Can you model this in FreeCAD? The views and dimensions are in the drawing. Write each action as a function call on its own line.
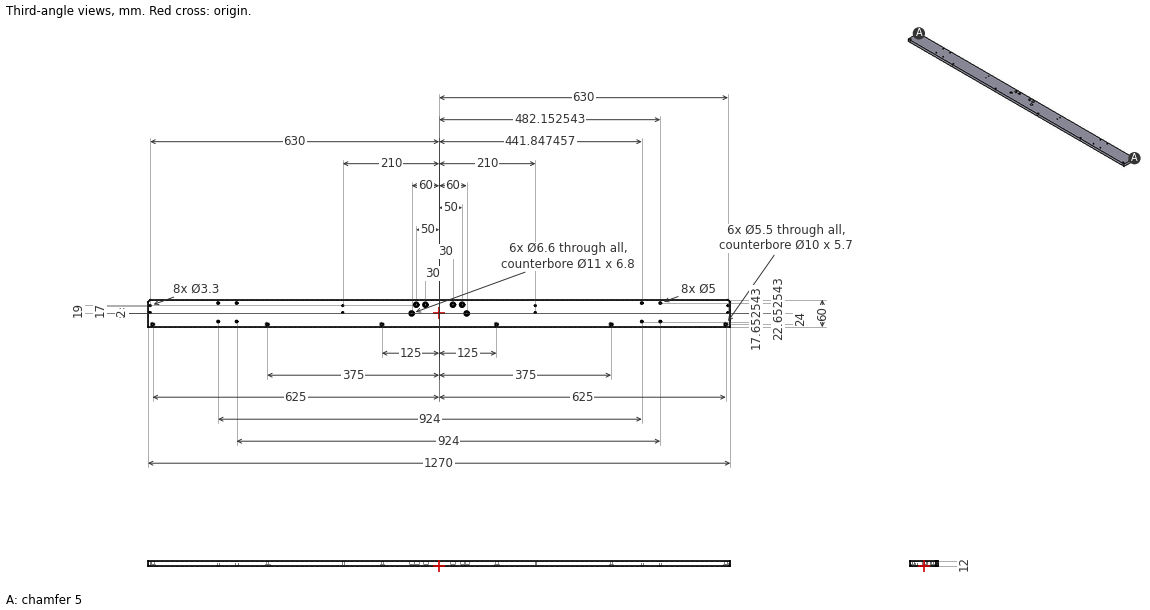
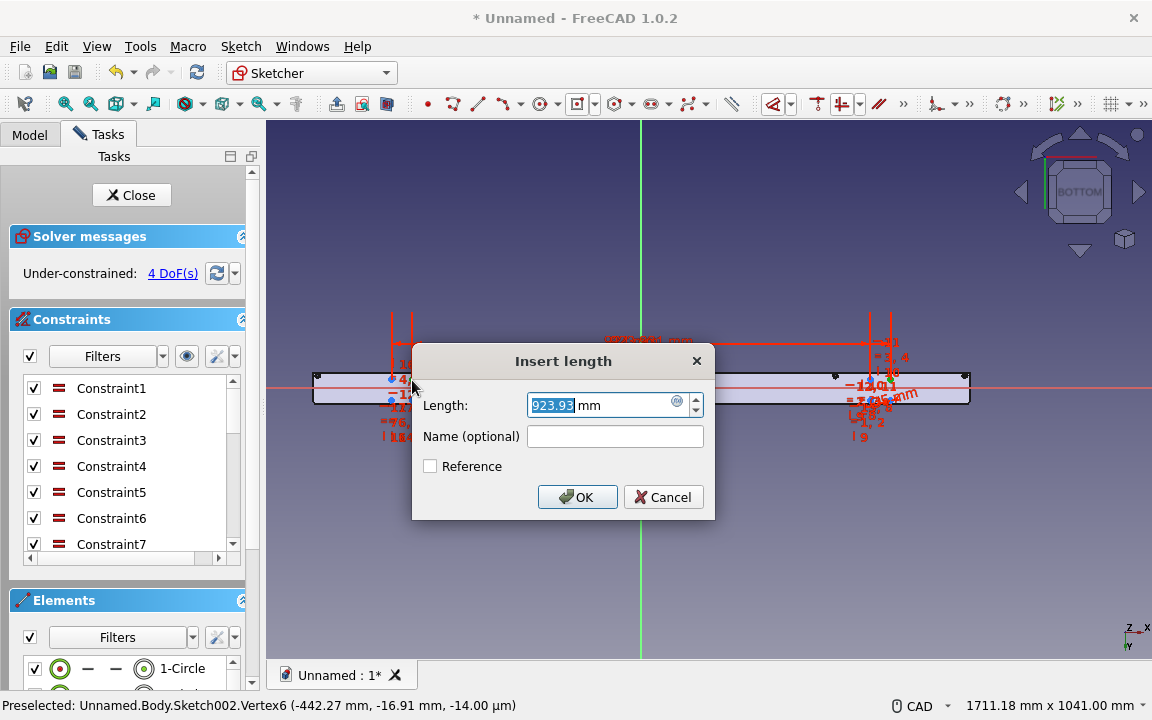
text(924)
key(Return)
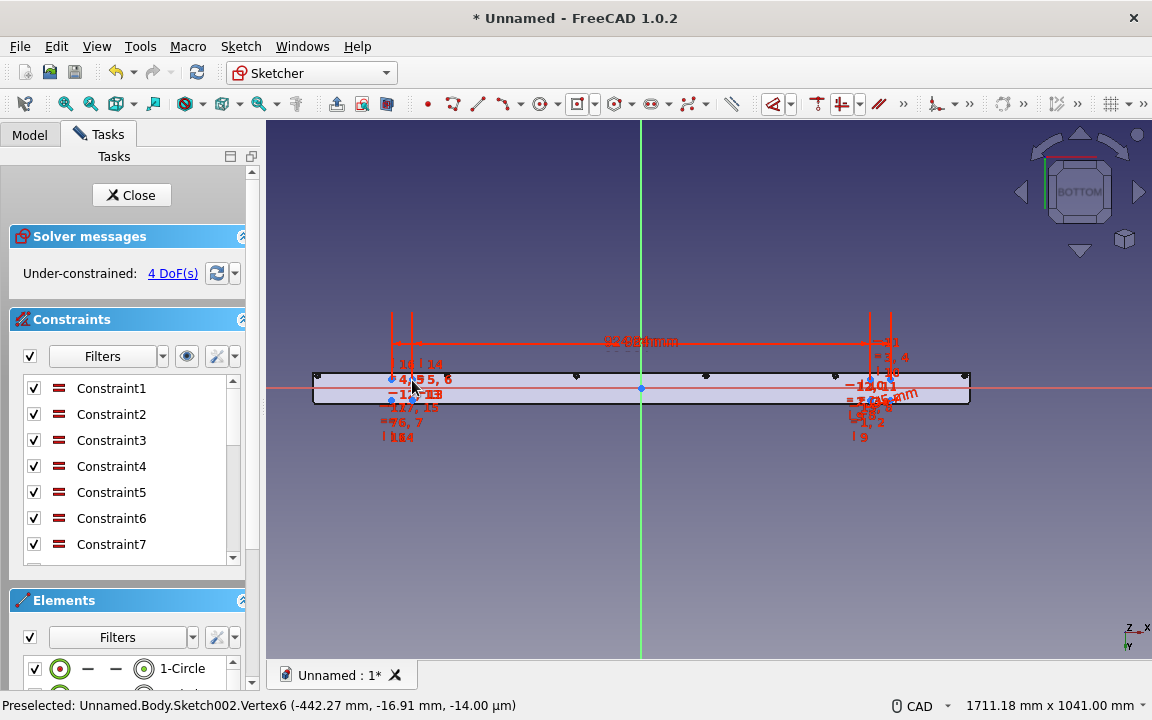
scroll(891, 401, up, 7)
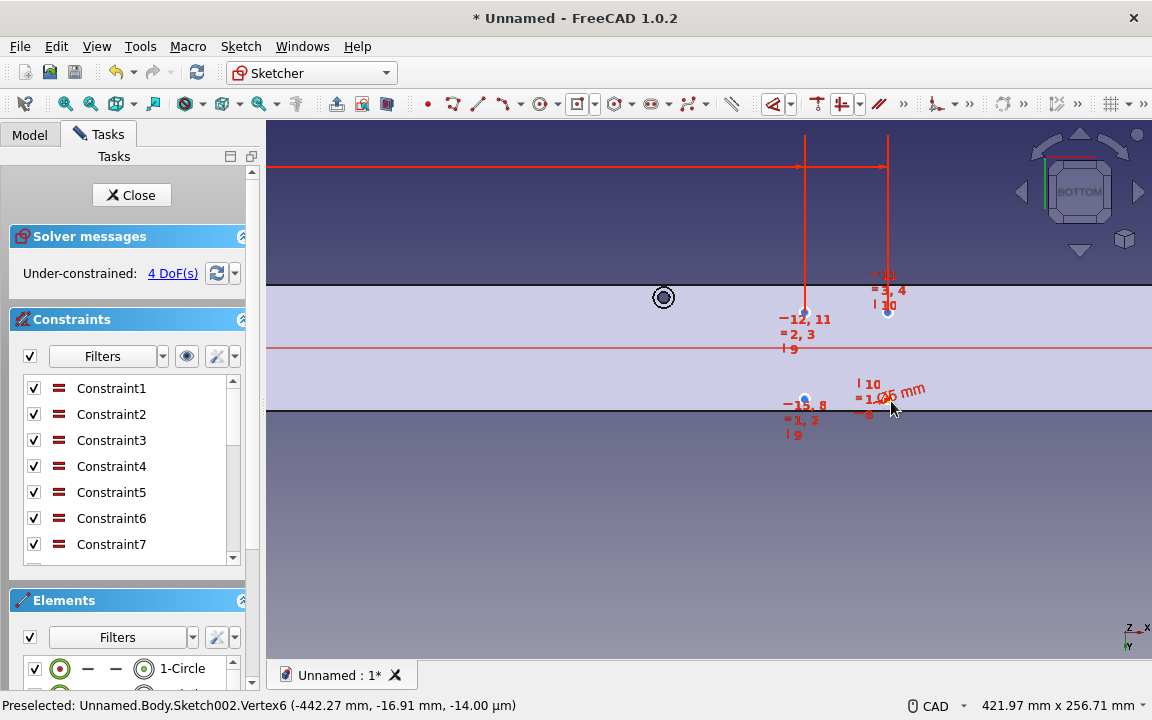
click(888, 399)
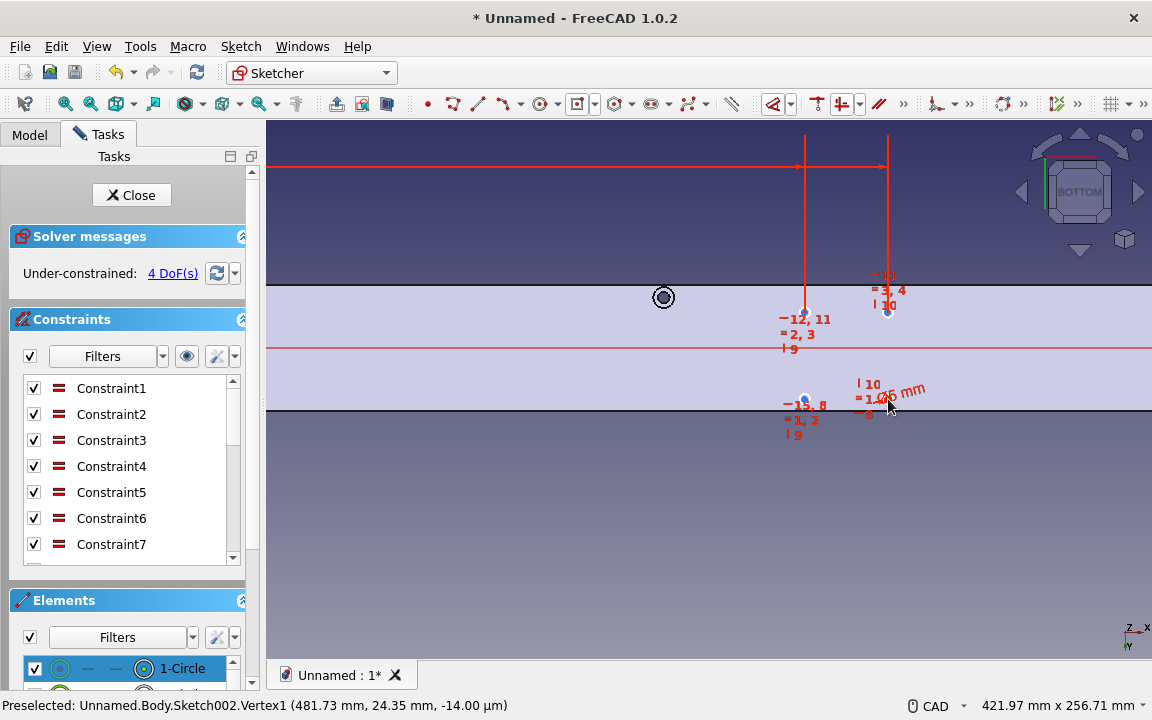
click(790, 104)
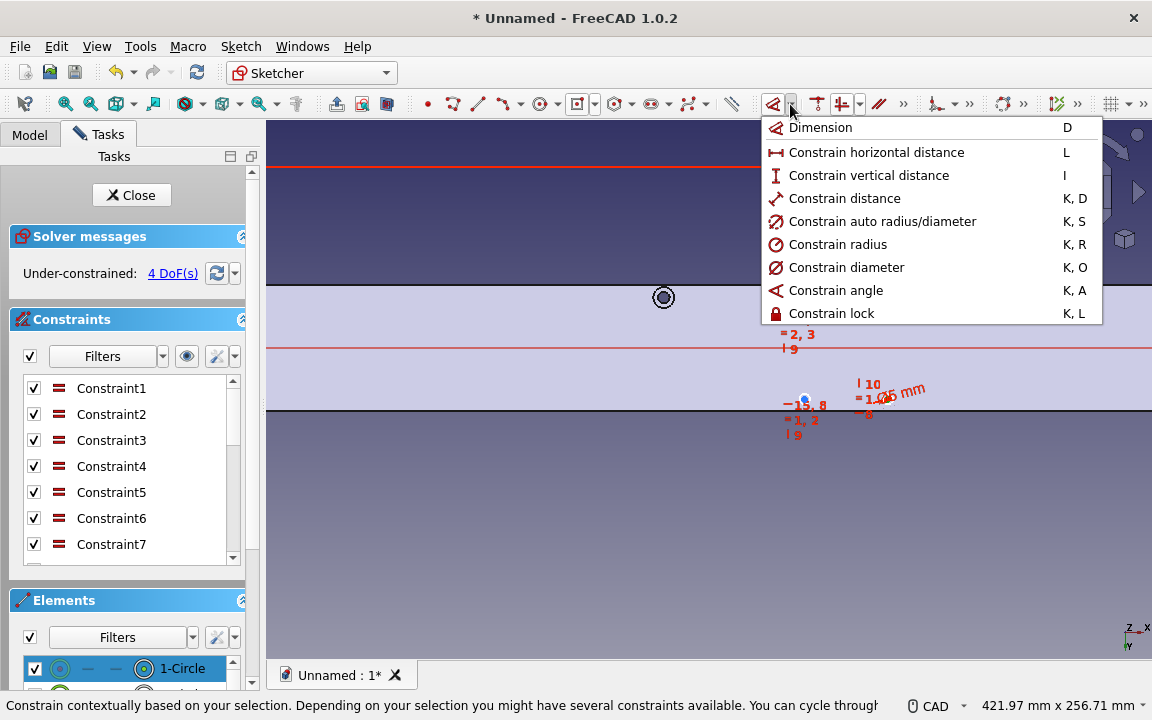
click(932, 176)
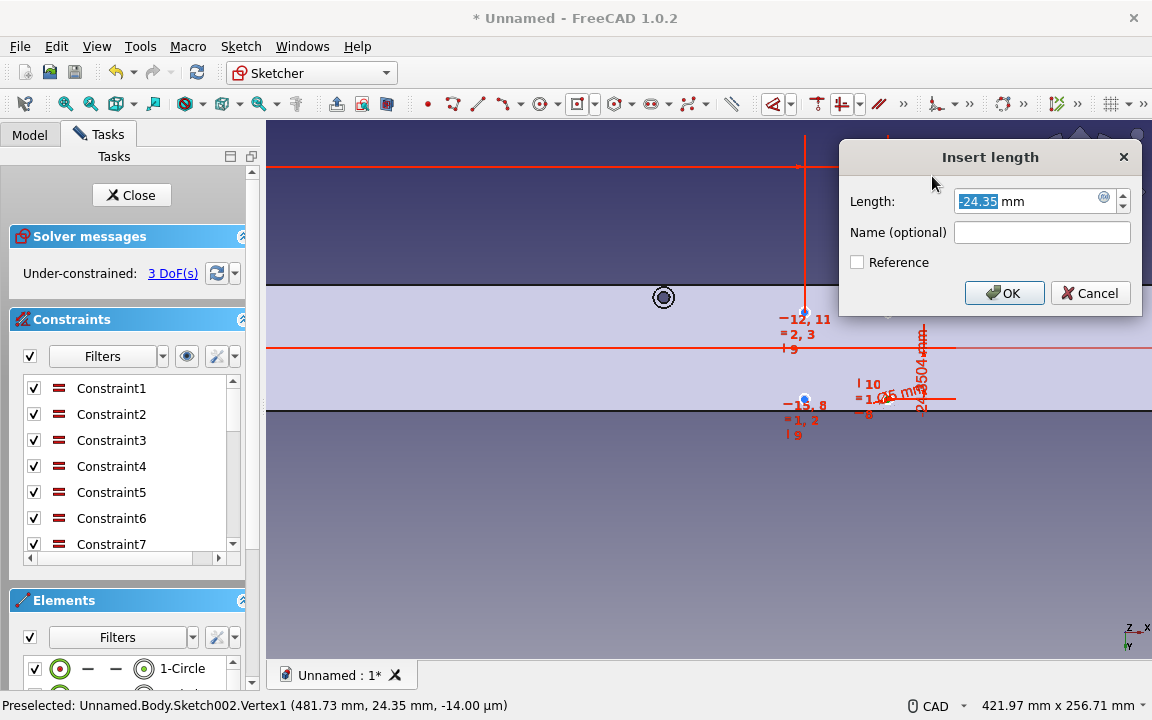
text(-22.652543)
key(Return)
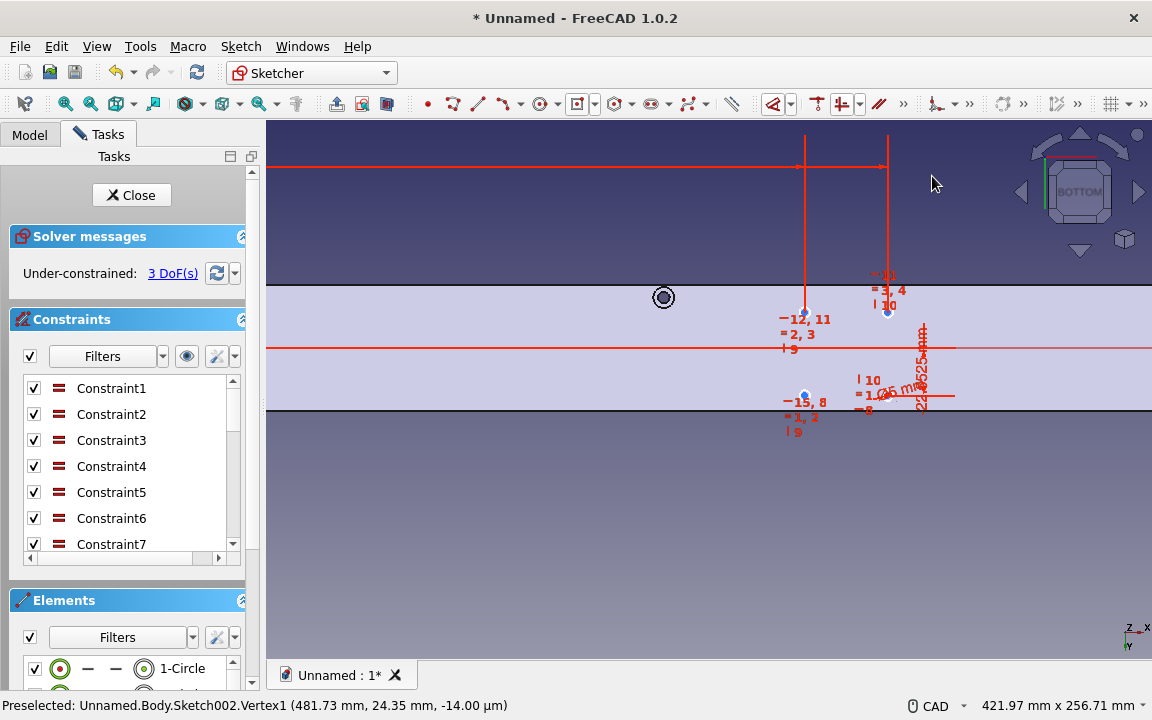
click(805, 312)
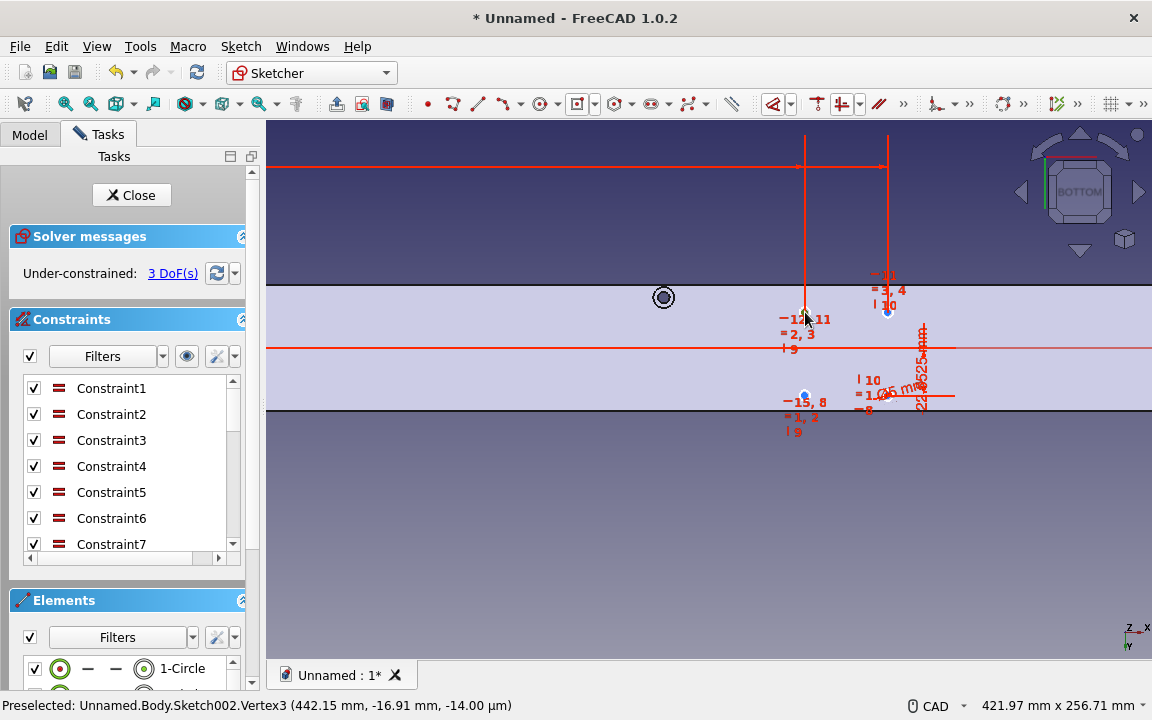
key(i)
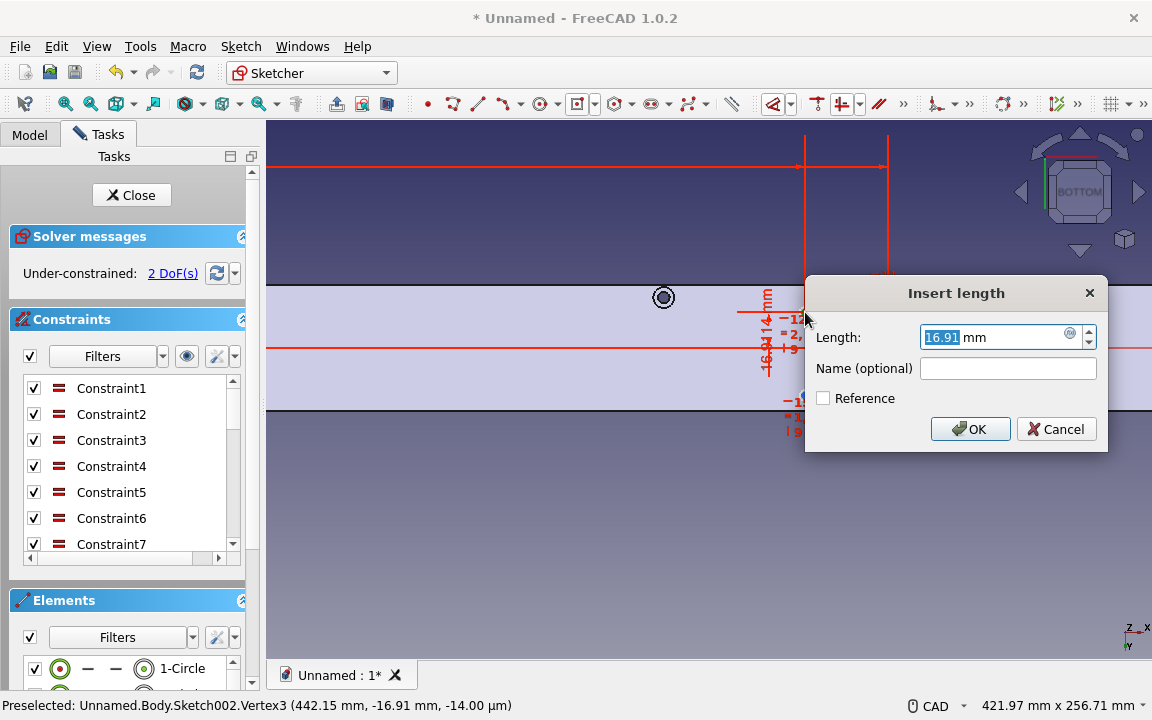
text(17.652543)
key(Return)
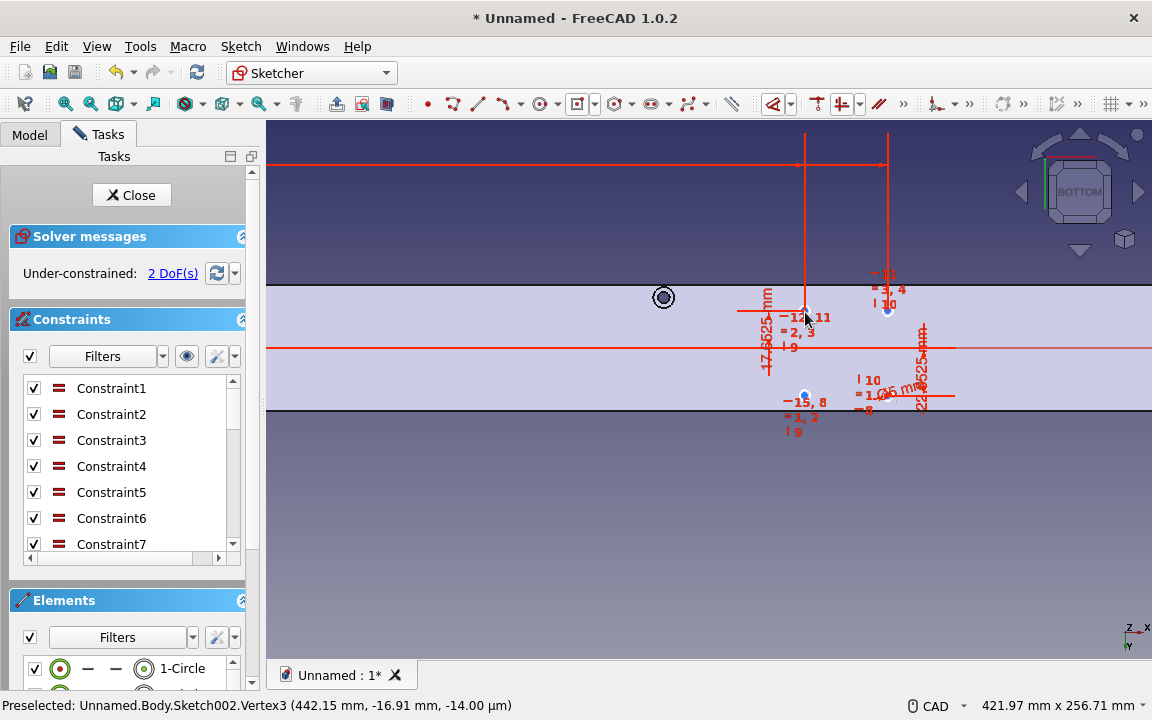
scroll(891, 401, down, 7)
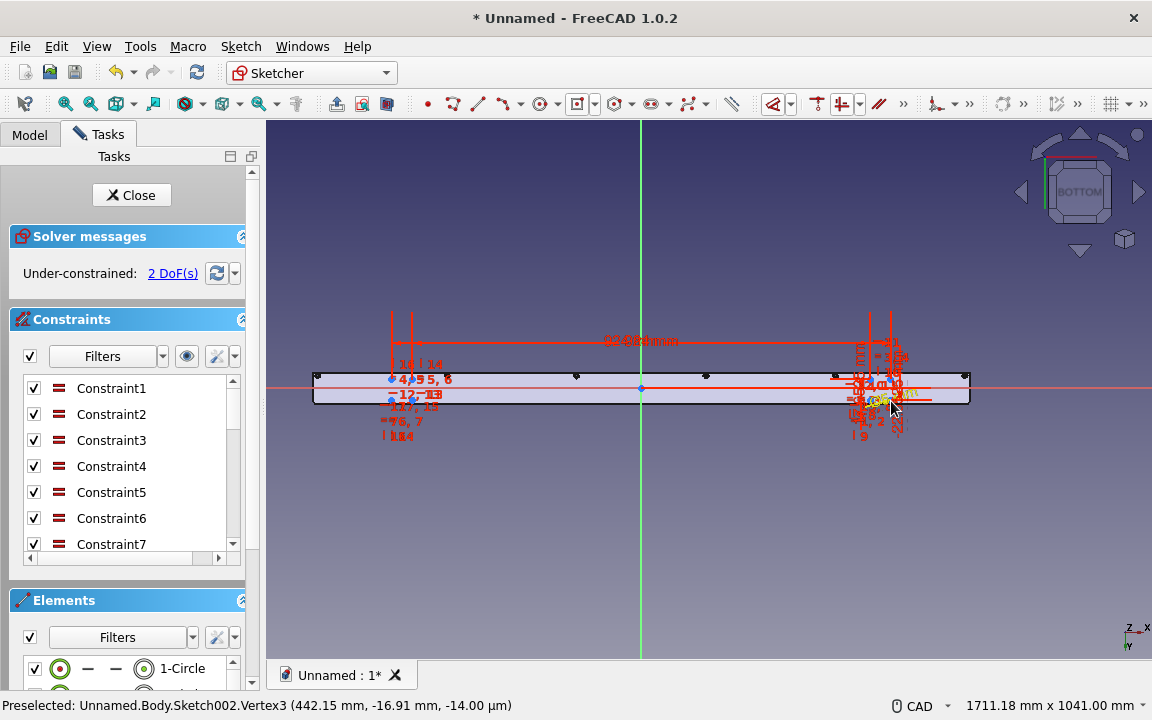
click(891, 400)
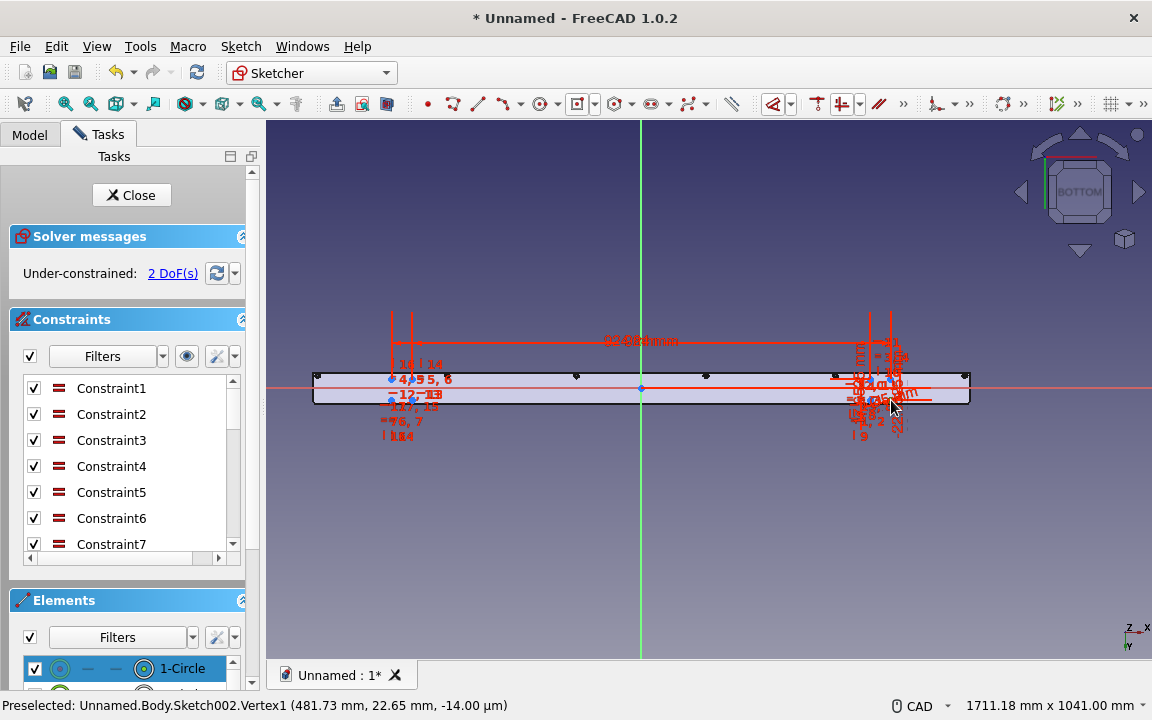
key(l)